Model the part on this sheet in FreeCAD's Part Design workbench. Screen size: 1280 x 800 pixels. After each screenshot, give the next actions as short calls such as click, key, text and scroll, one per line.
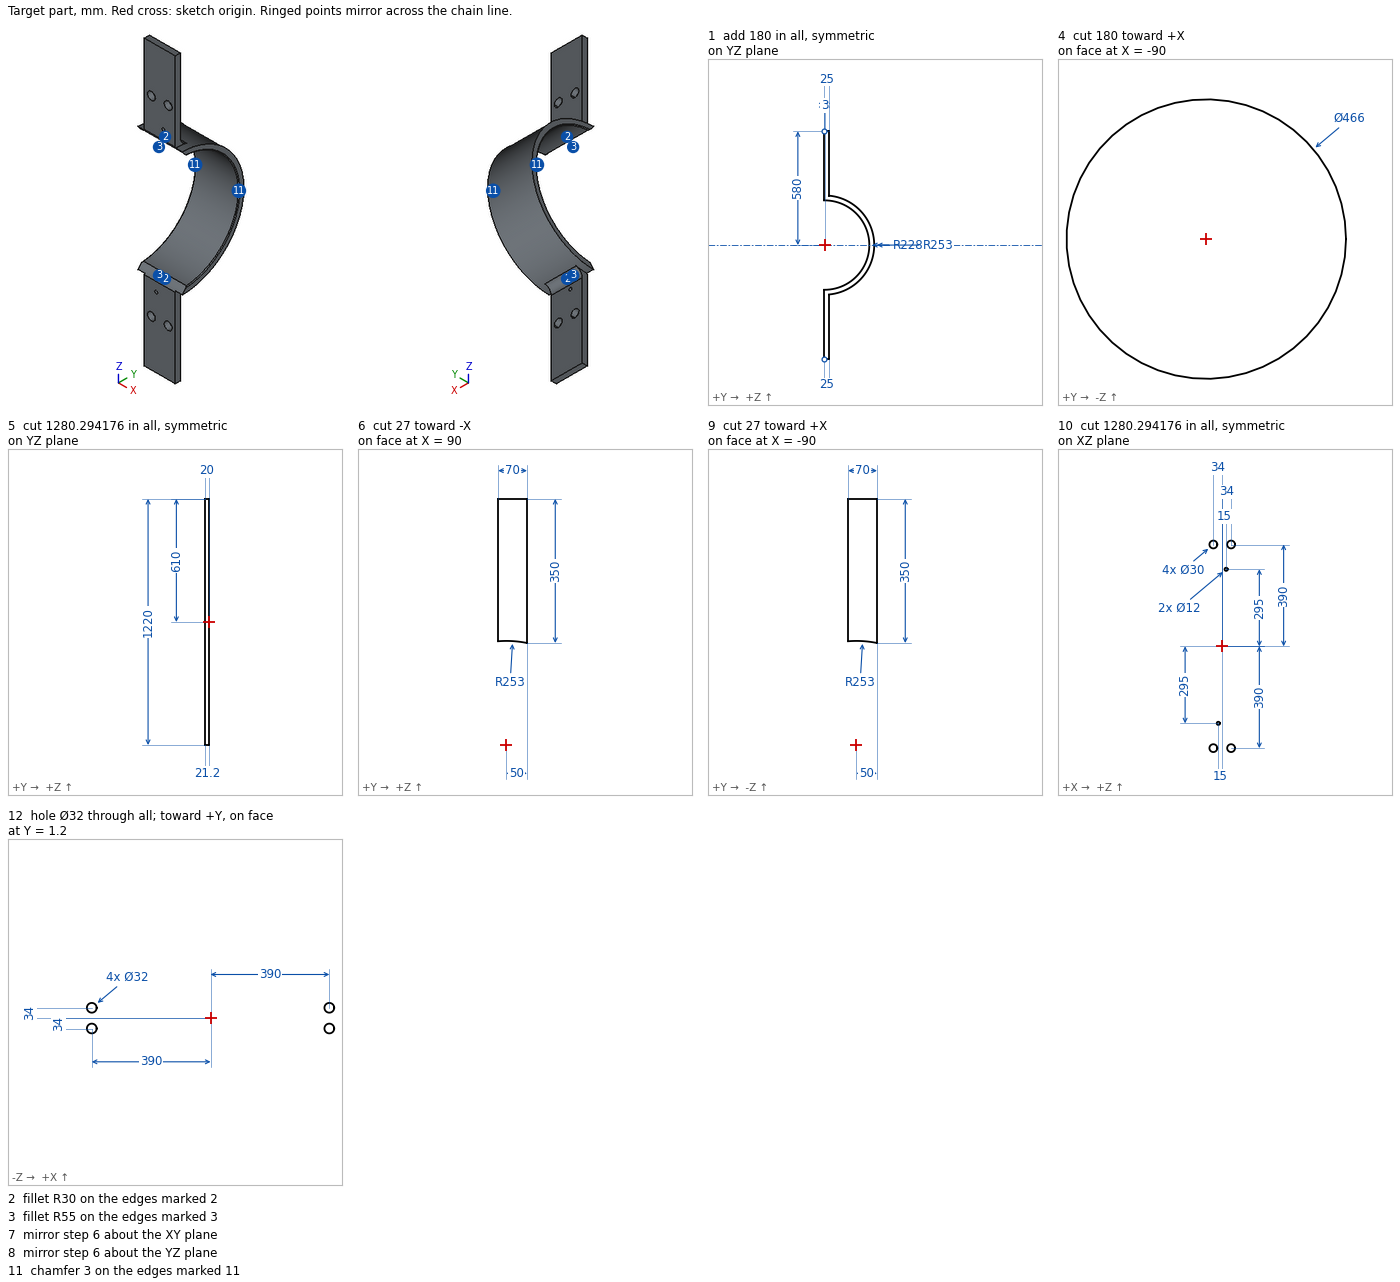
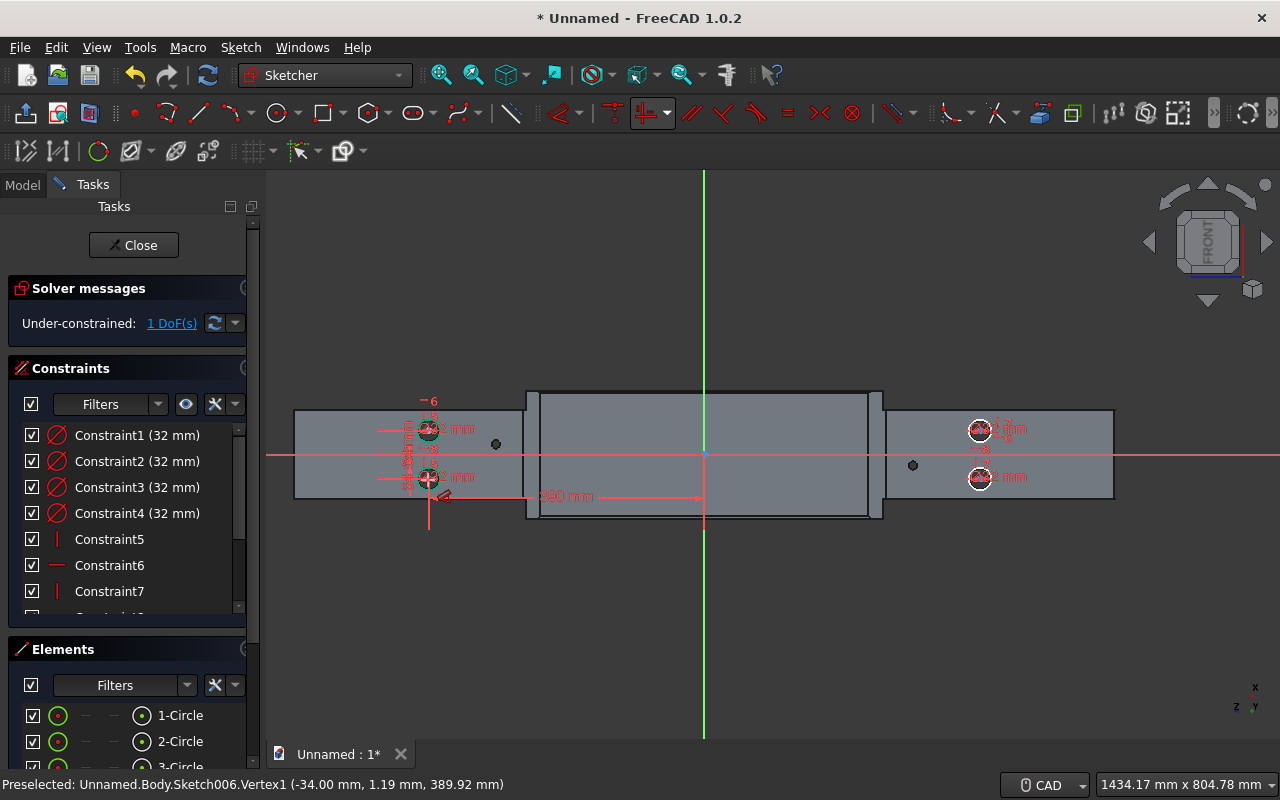
click(980, 431)
click(842, 397)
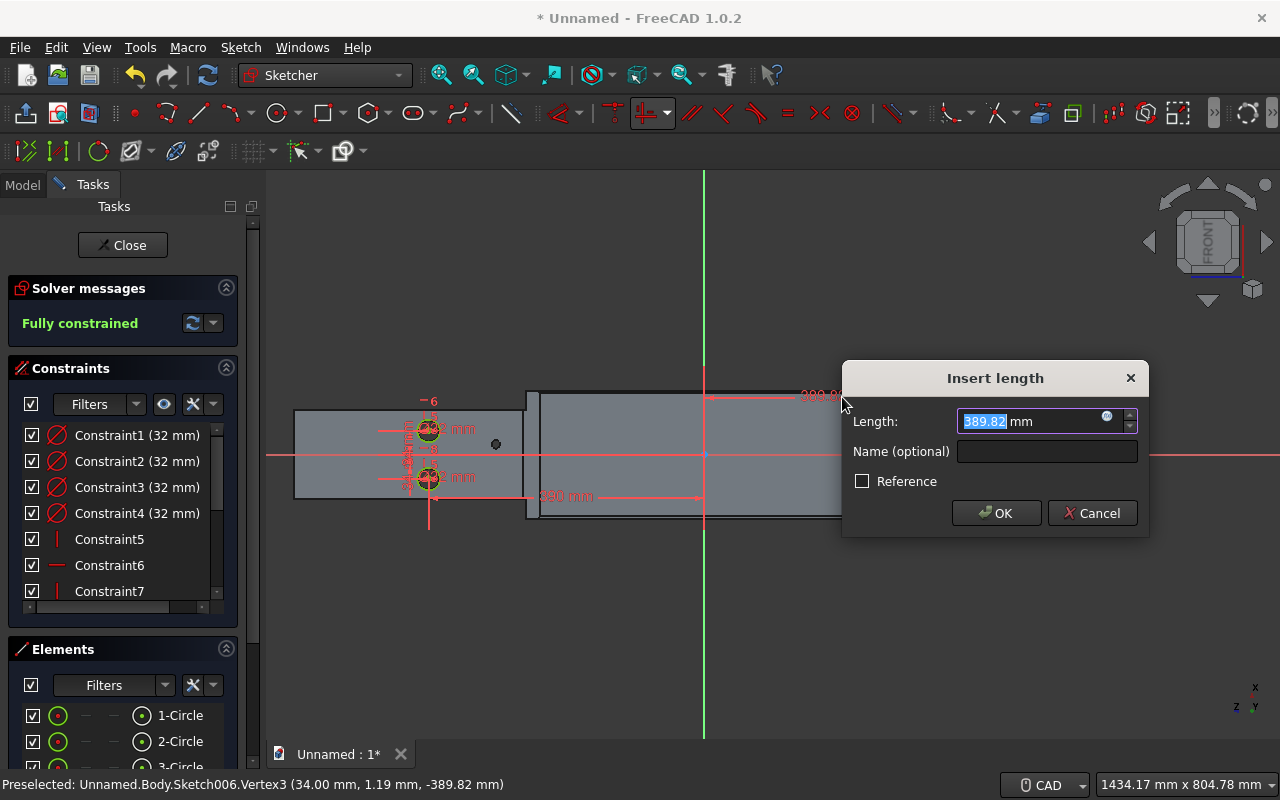
text(390)
key(Return)
key(Escape)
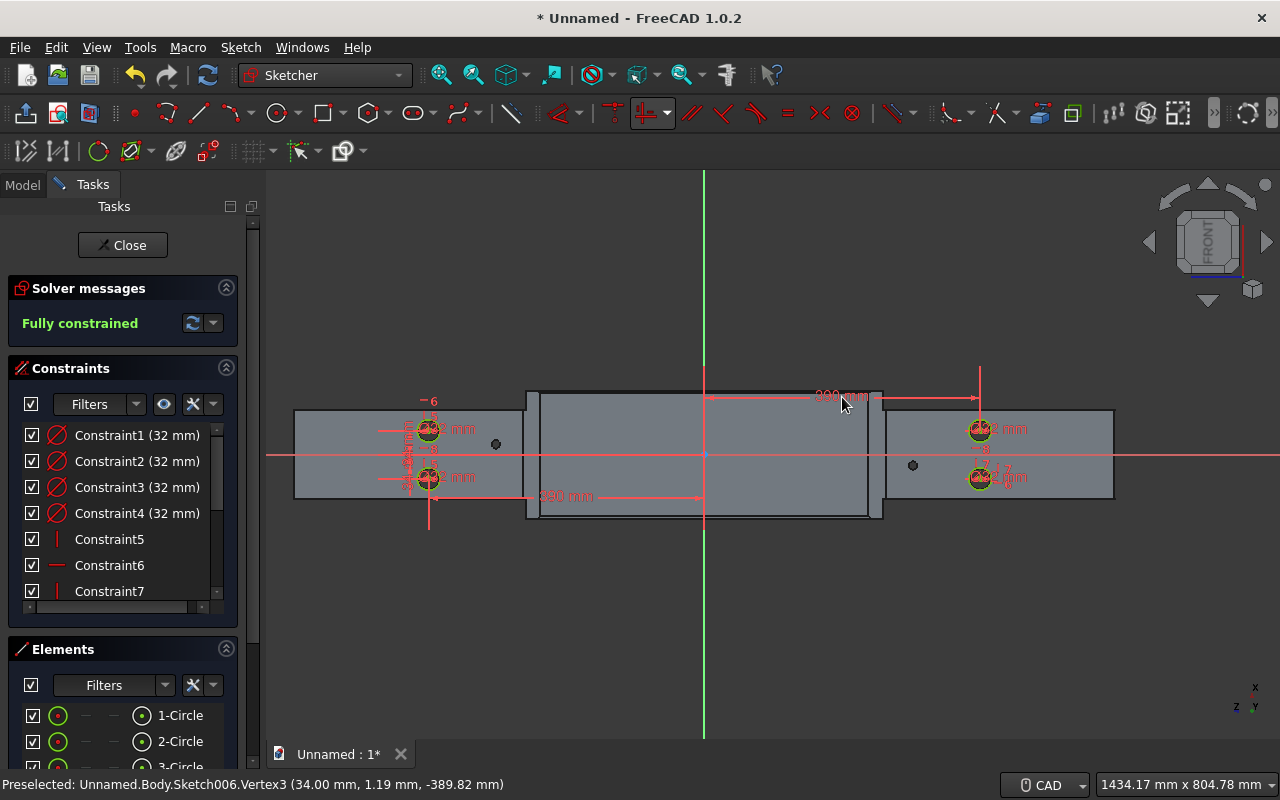
click(123, 245)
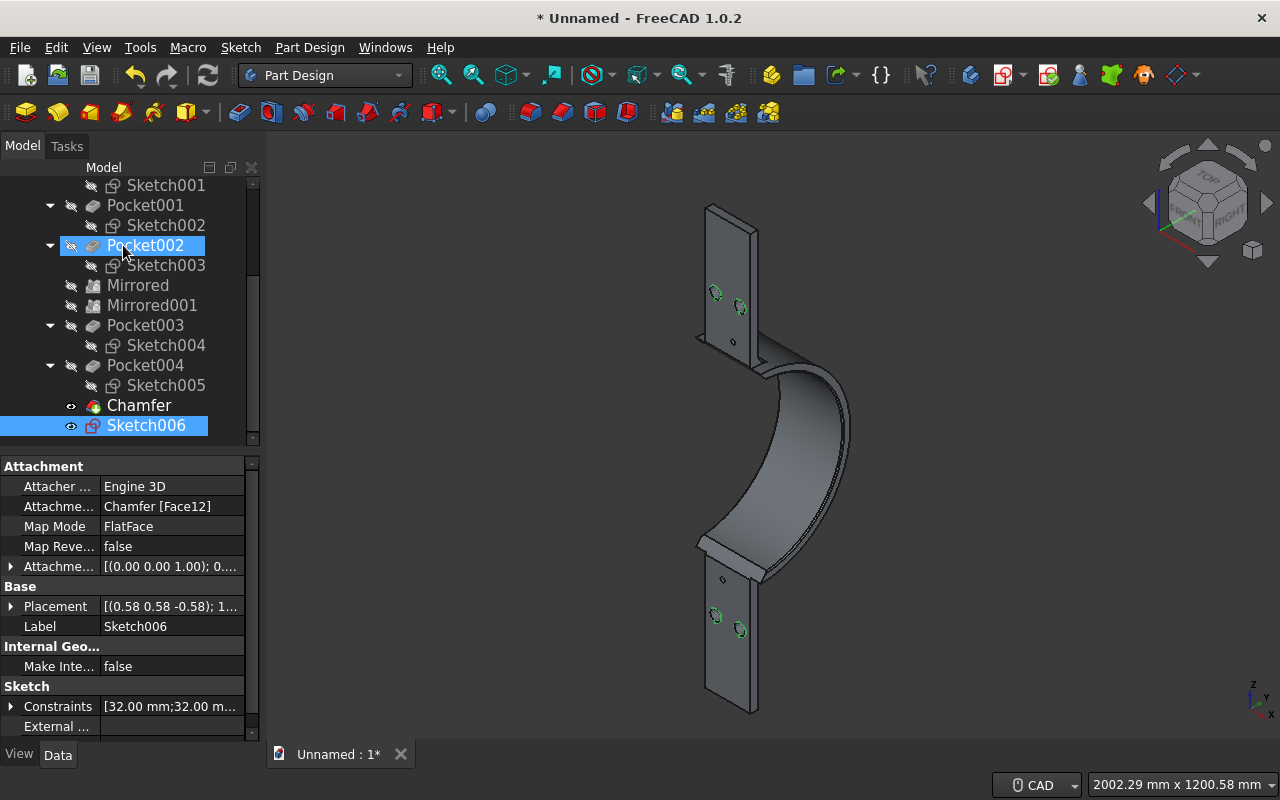
click(272, 112)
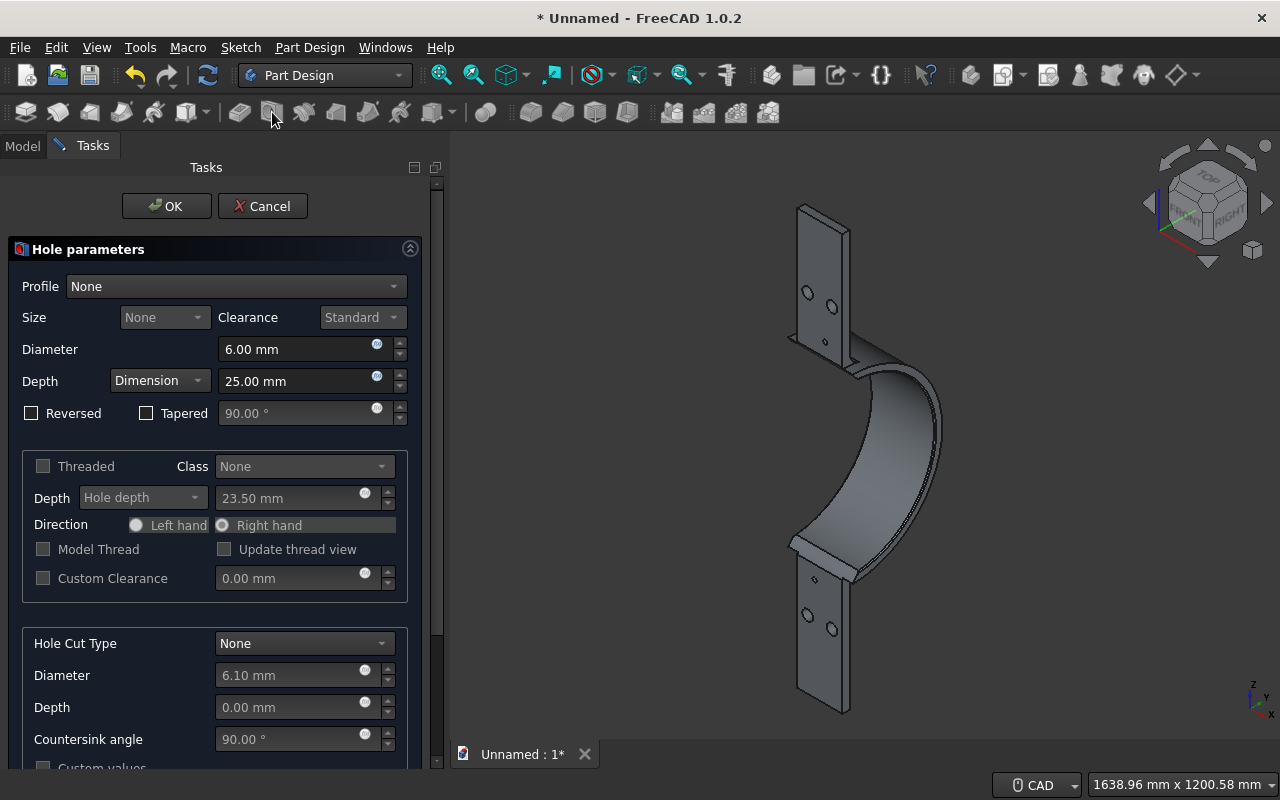
triple_click(305, 349)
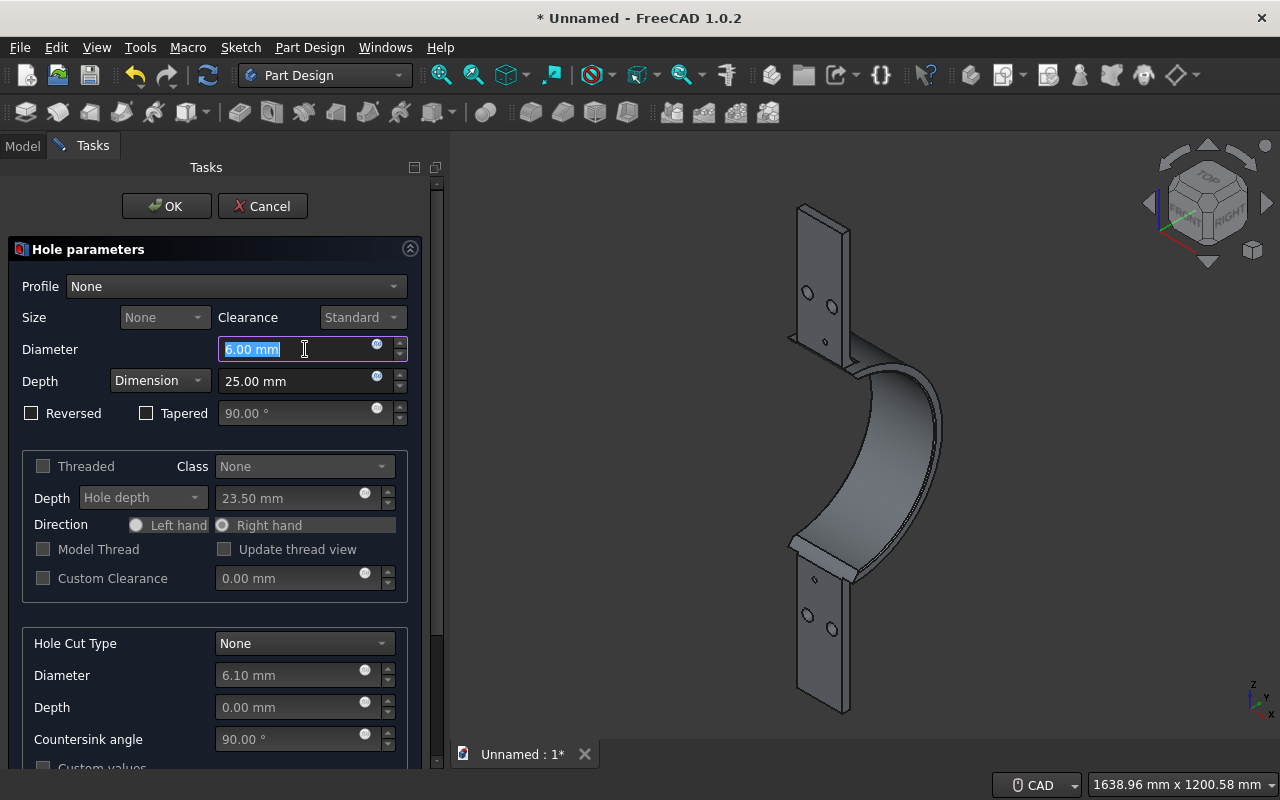
text(32)
key(Tab)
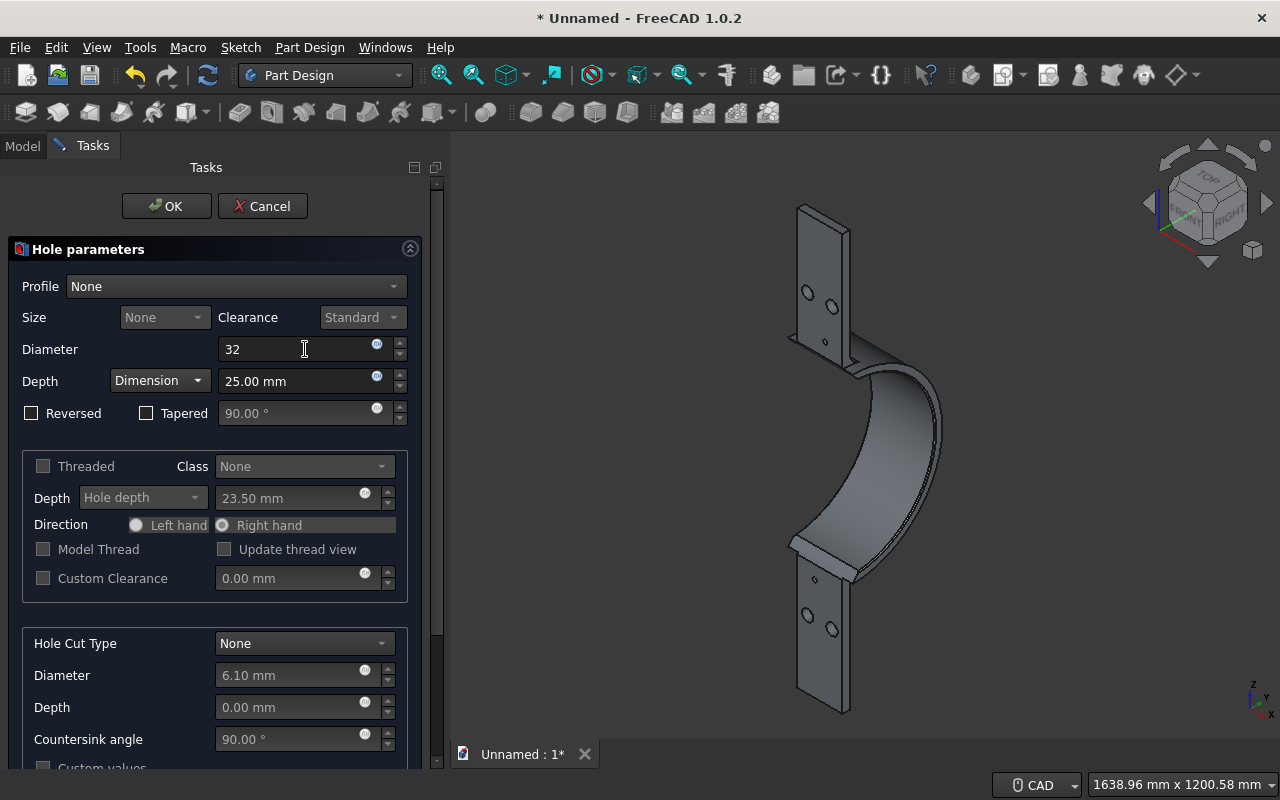
click(161, 380)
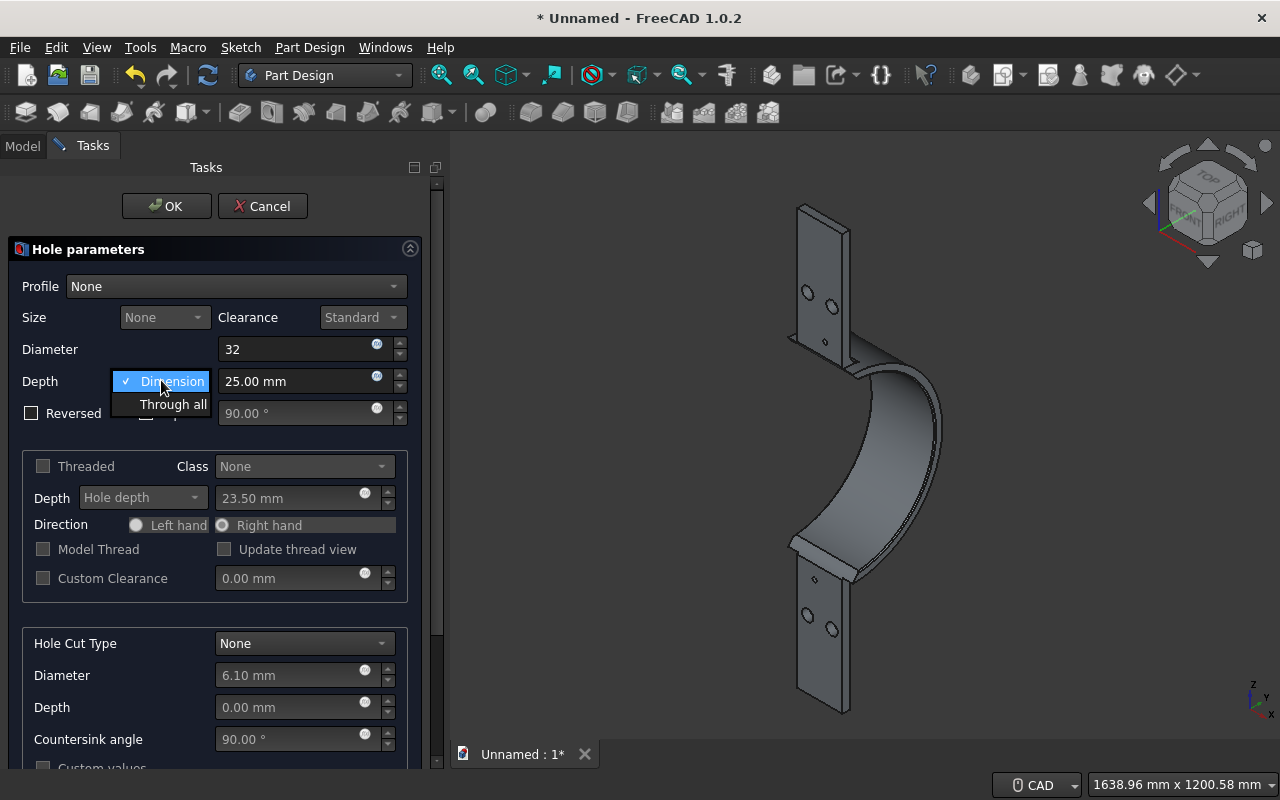
click(160, 404)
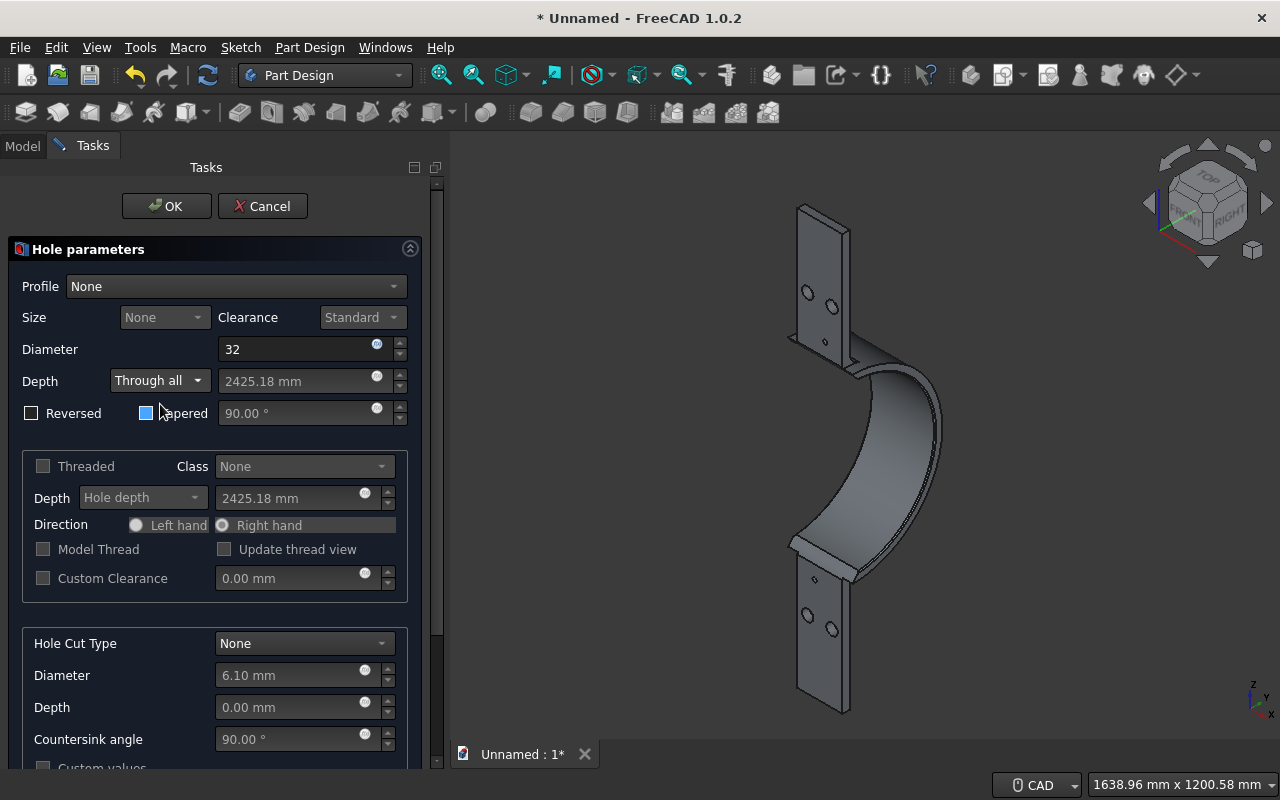
click(167, 206)